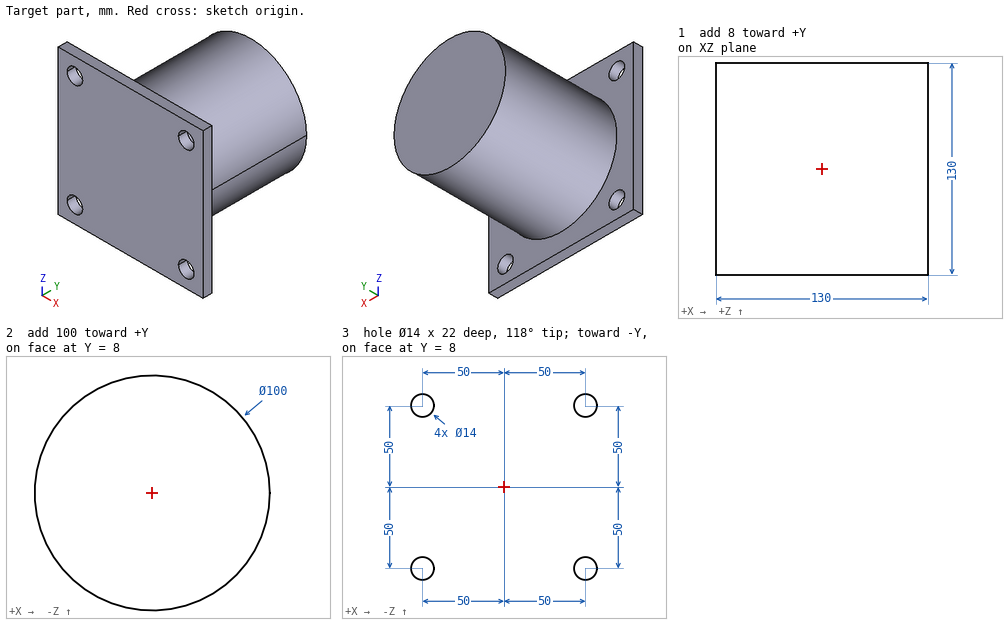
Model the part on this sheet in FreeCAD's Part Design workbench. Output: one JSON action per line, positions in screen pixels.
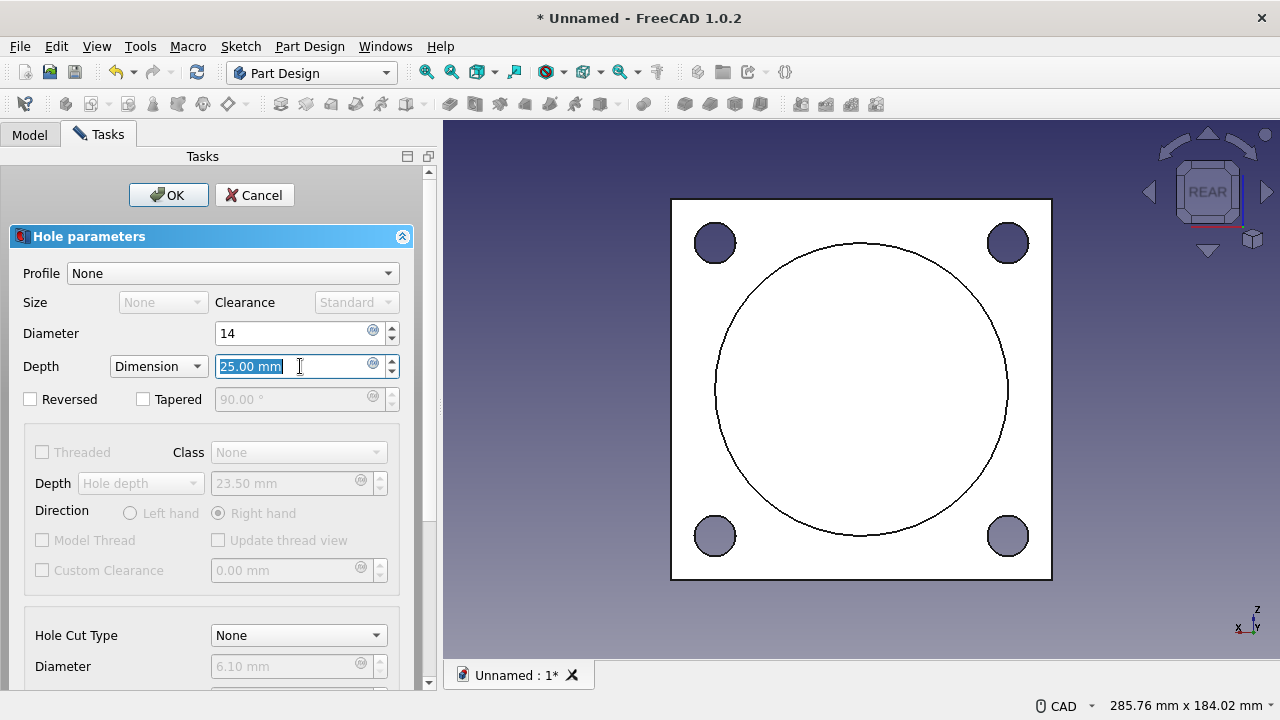
{"action": "type", "text": "22"}
{"action": "key", "text": "Tab"}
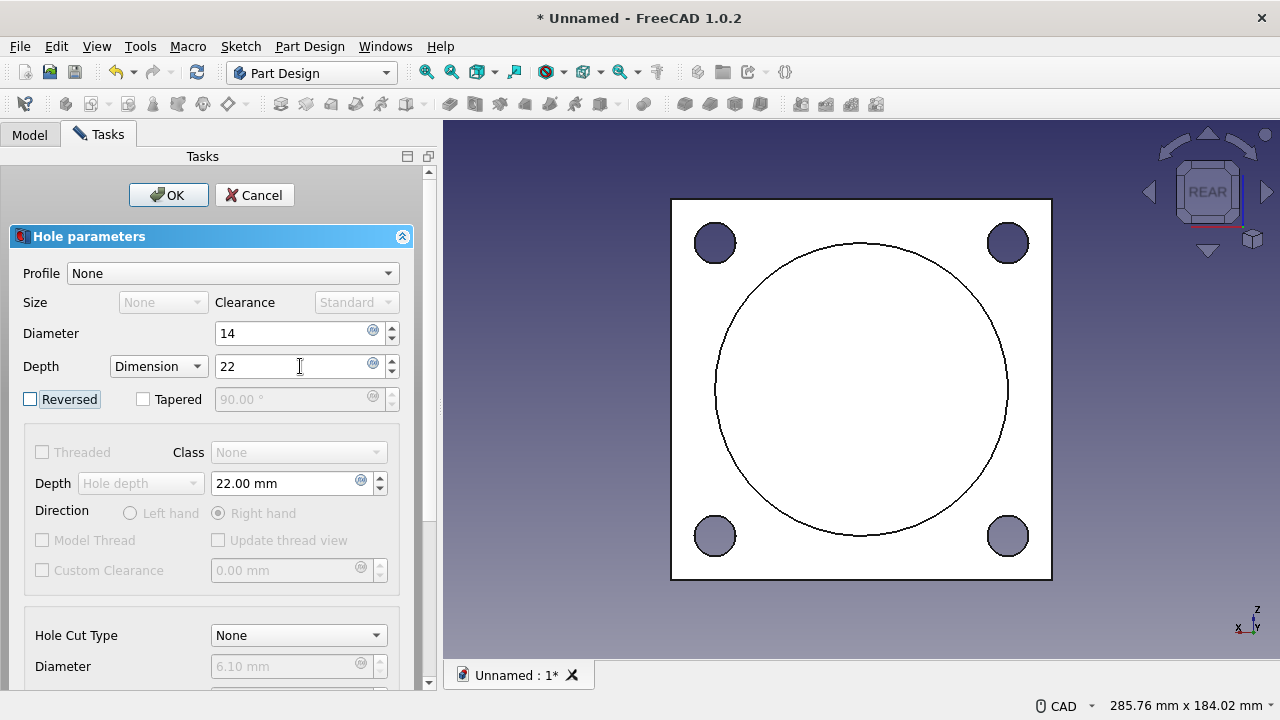
{"action": "left_click", "coordinate": [169, 195]}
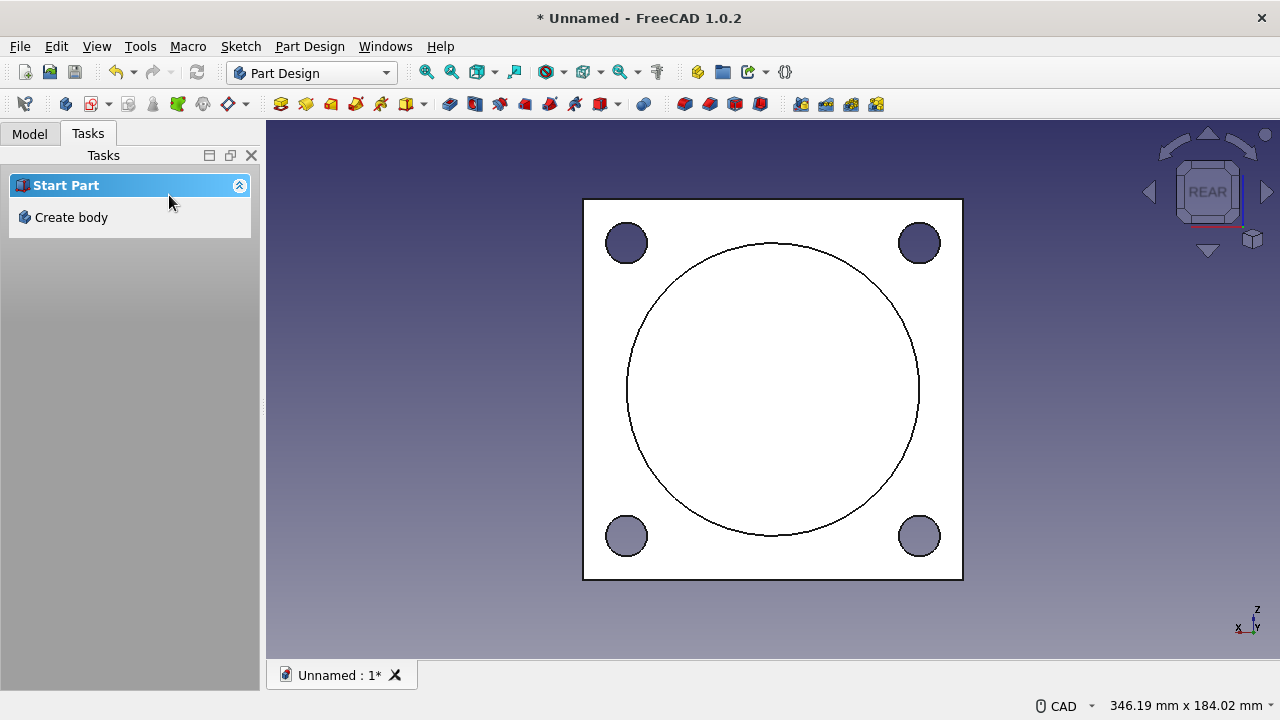
{"action": "key", "text": "0"}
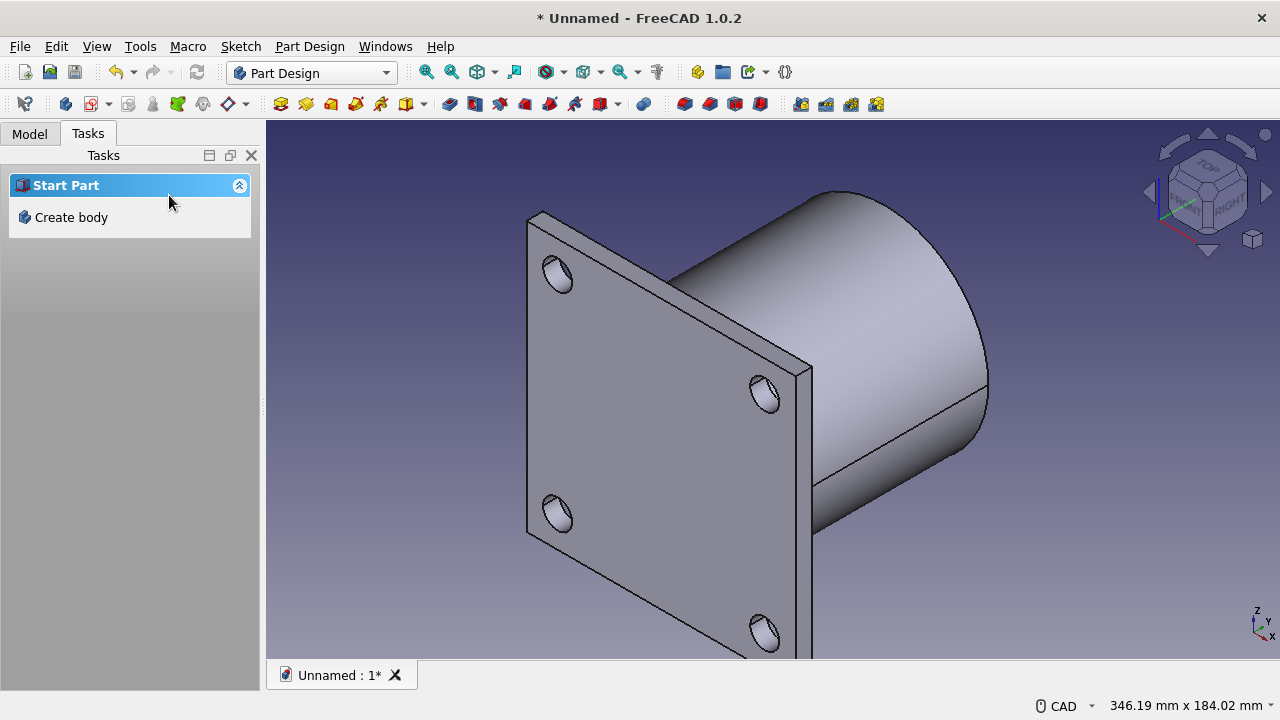
{"action": "left_click", "coordinate": [427, 72]}